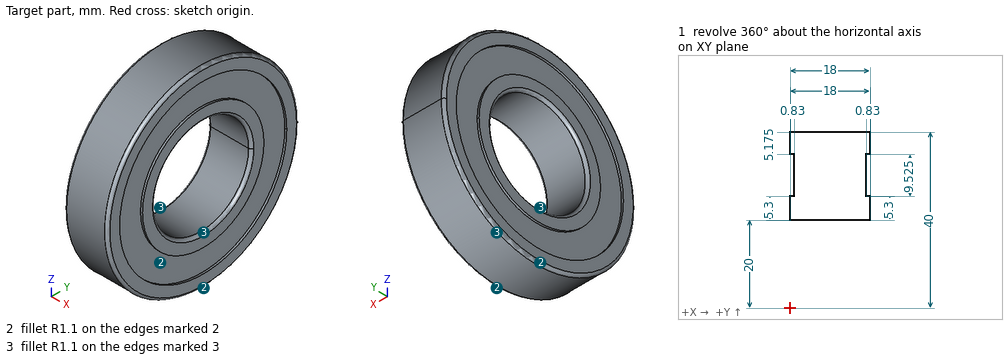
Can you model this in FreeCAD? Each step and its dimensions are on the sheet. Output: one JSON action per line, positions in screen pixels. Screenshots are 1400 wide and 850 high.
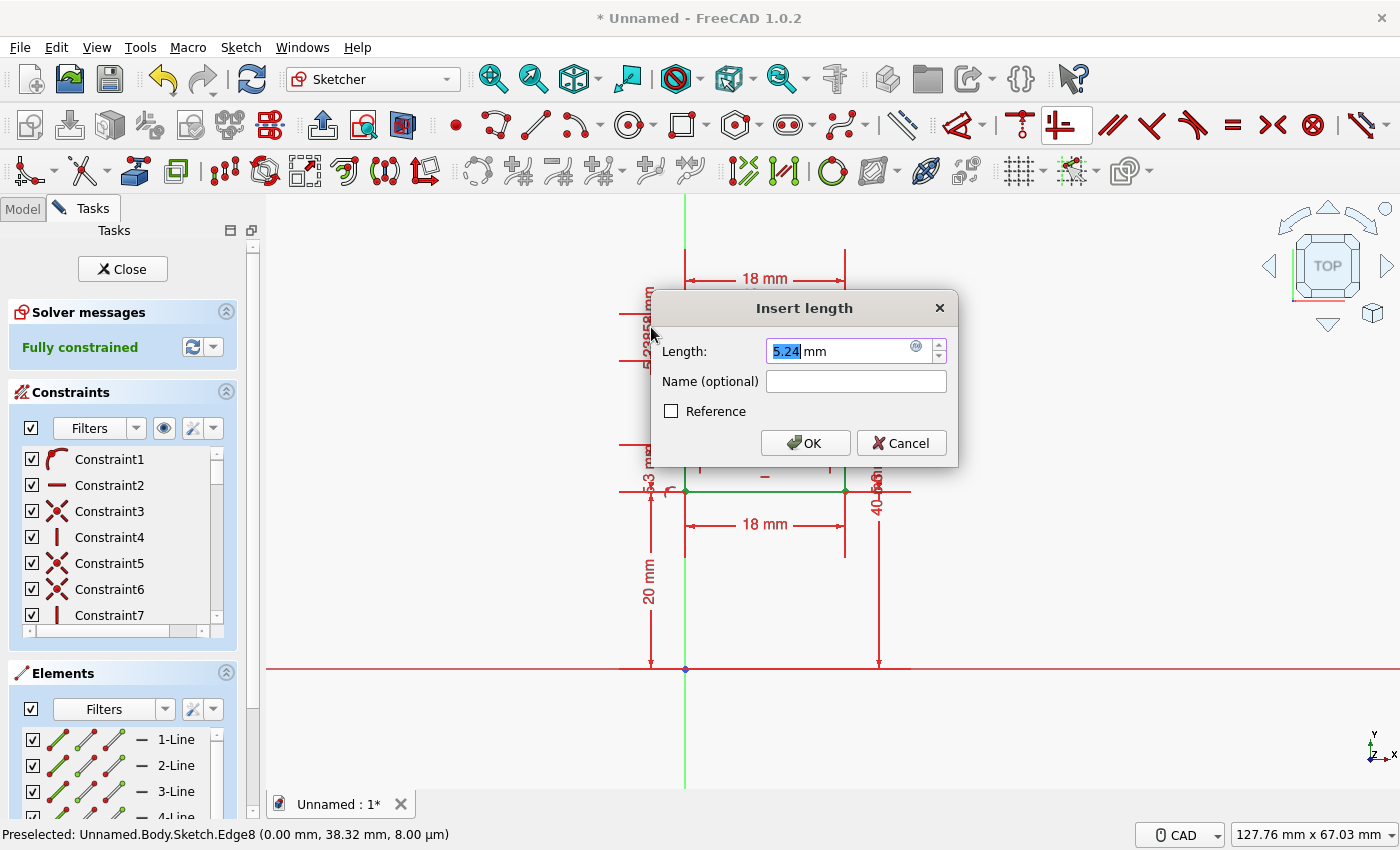
{"action": "type", "text": "5.175"}
{"action": "key", "text": "Return"}
{"action": "key", "text": "Escape"}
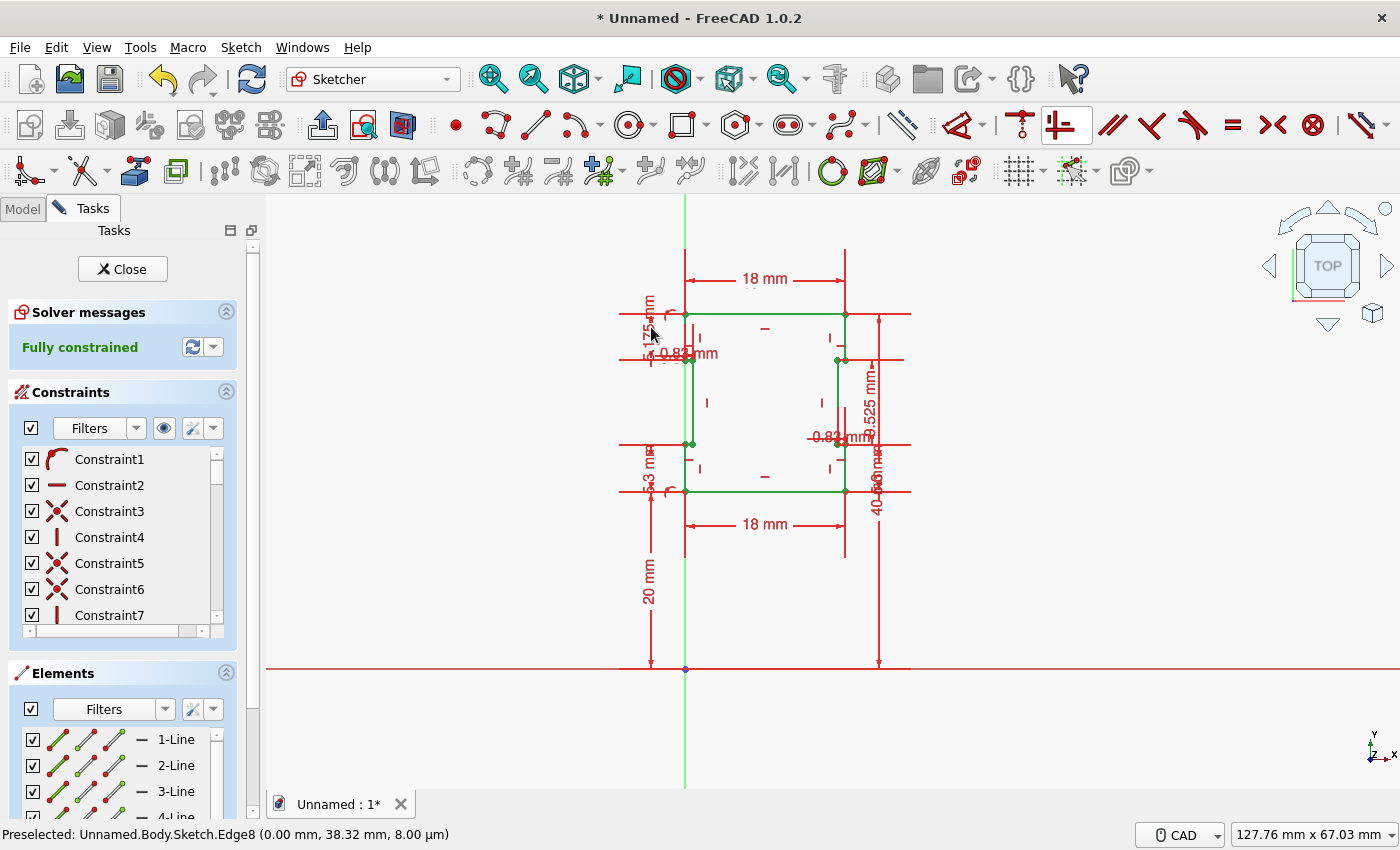
{"action": "left_click", "coordinate": [123, 269]}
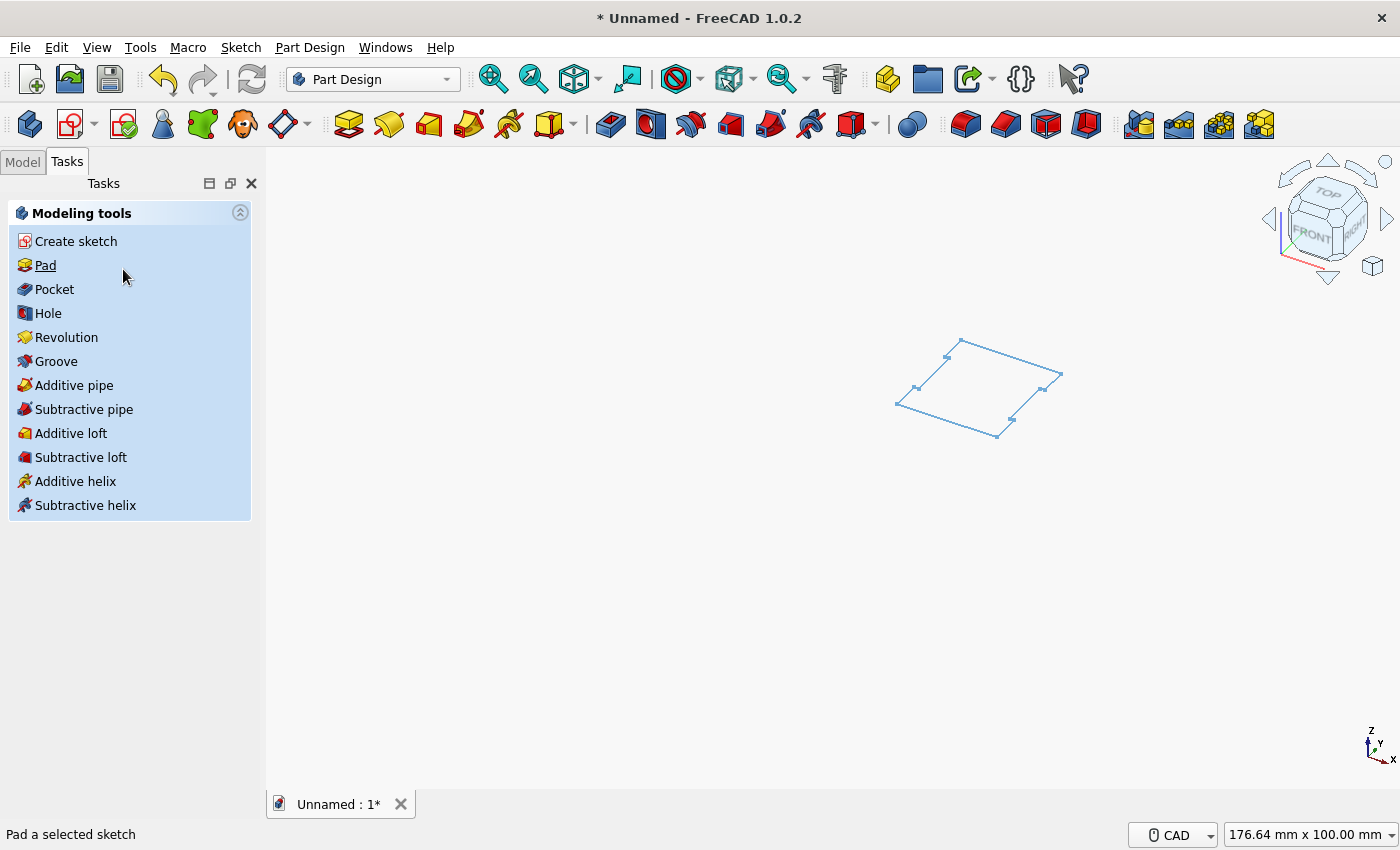
{"action": "left_click", "coordinate": [390, 124]}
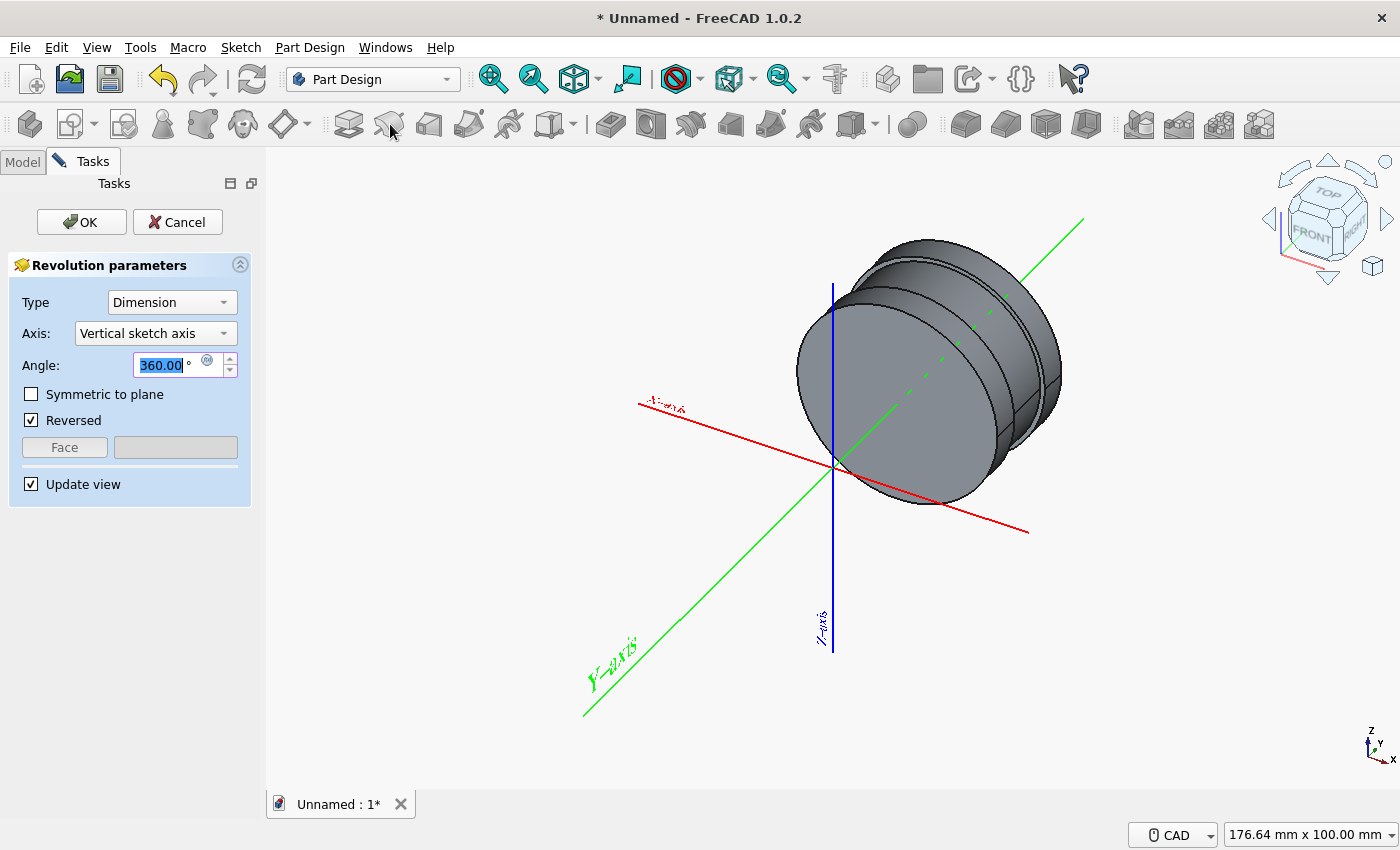
{"action": "left_click", "coordinate": [156, 334]}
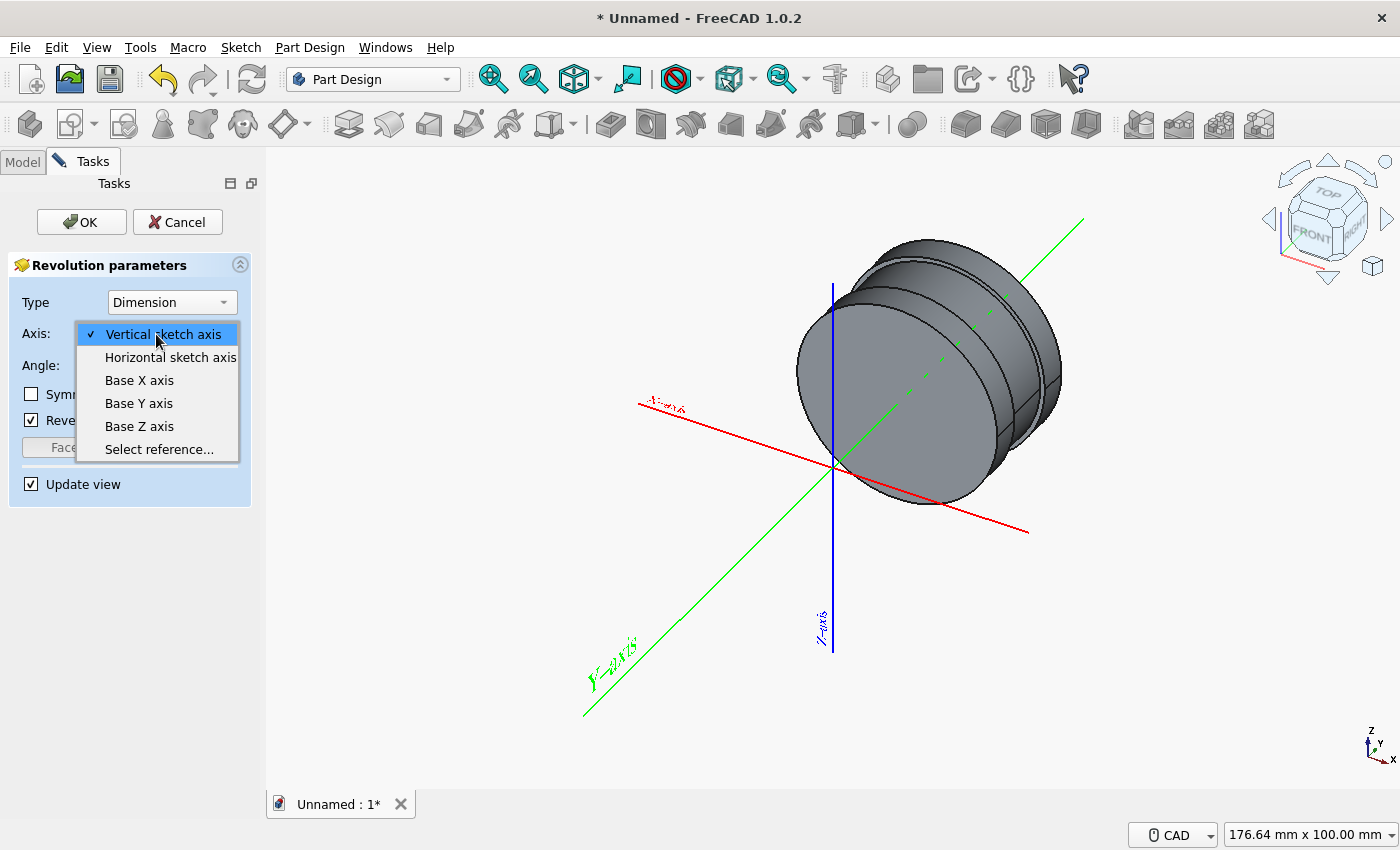
{"action": "left_click", "coordinate": [156, 358]}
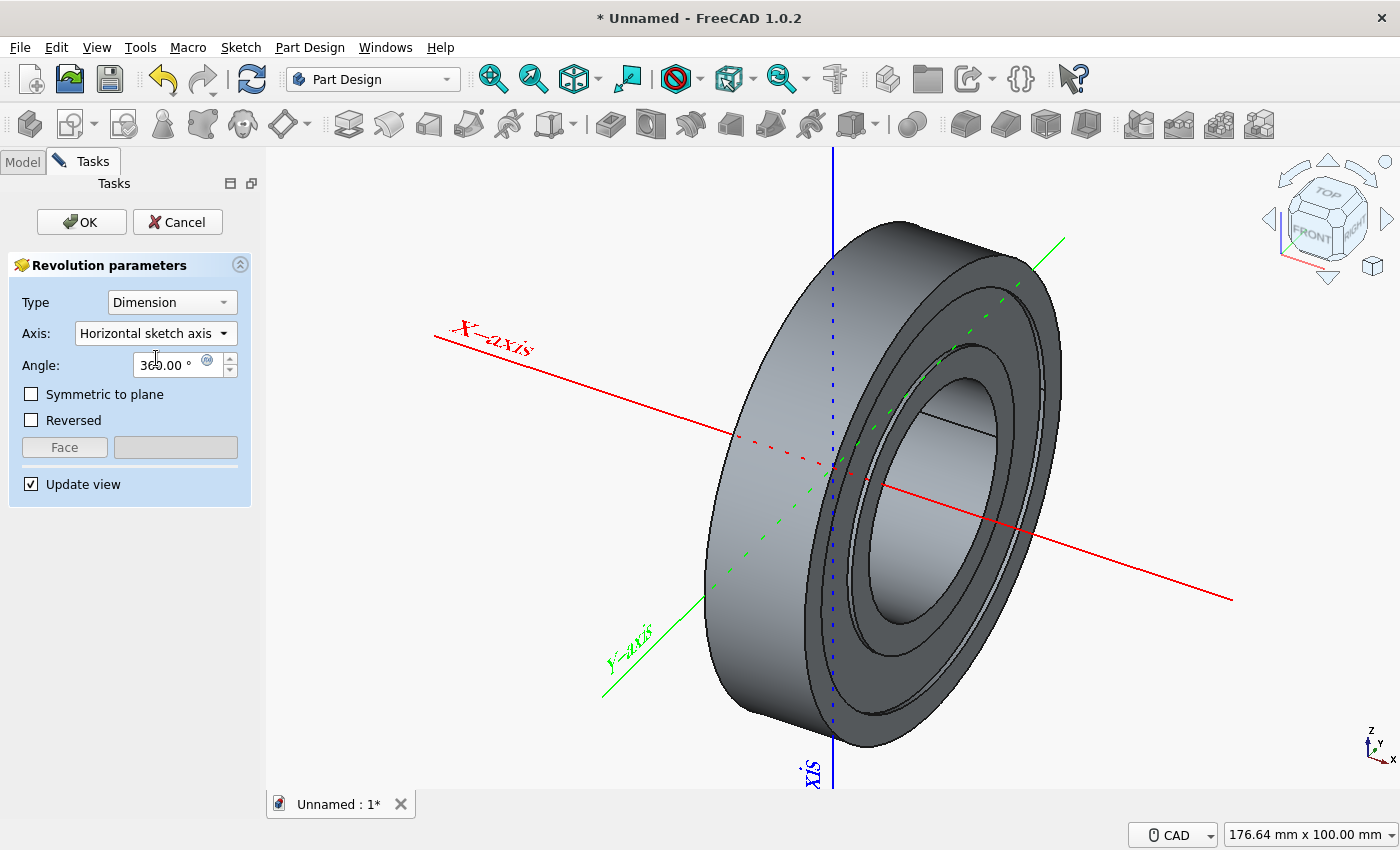
{"action": "left_click", "coordinate": [82, 222]}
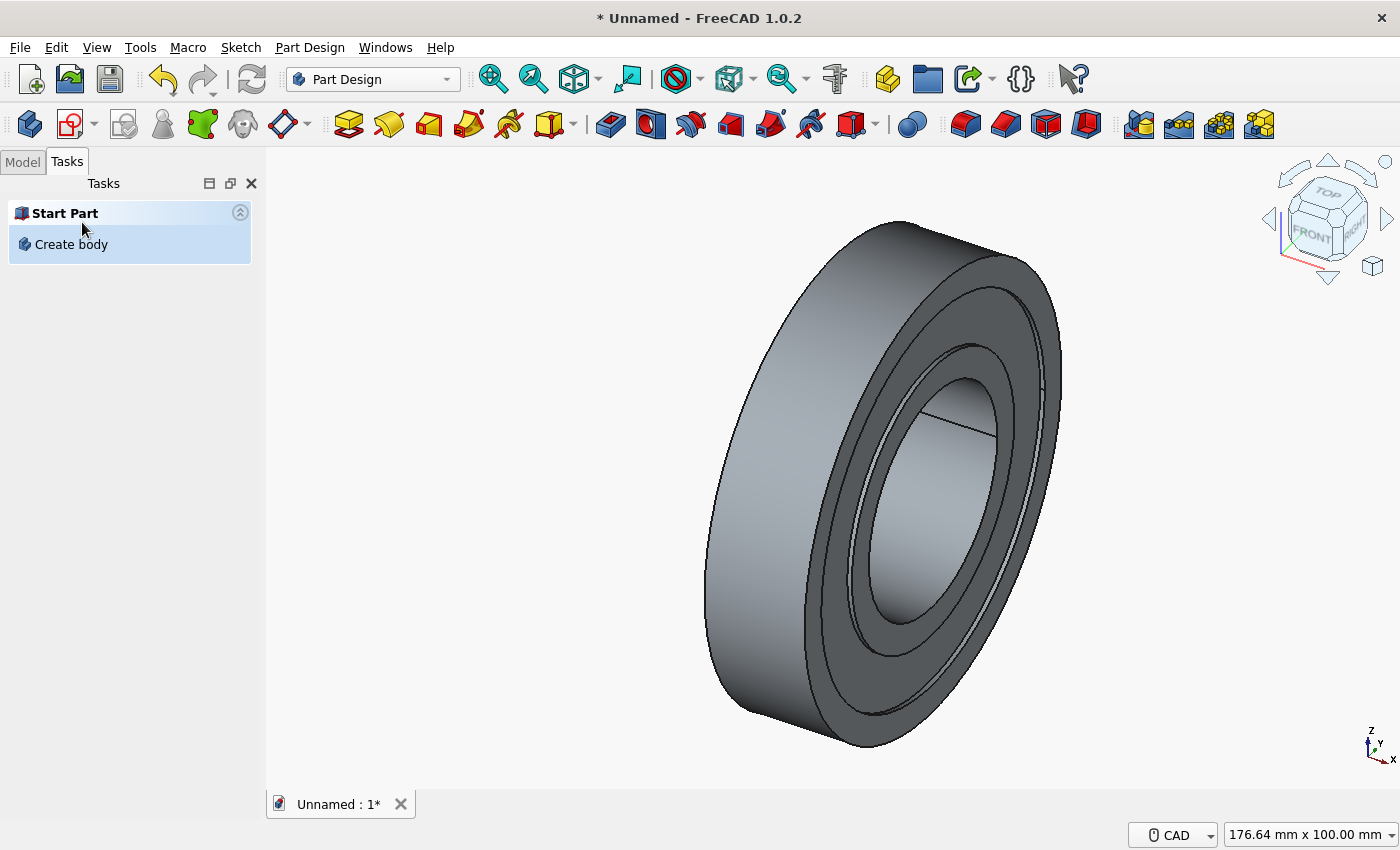
{"action": "left_click", "coordinate": [494, 80]}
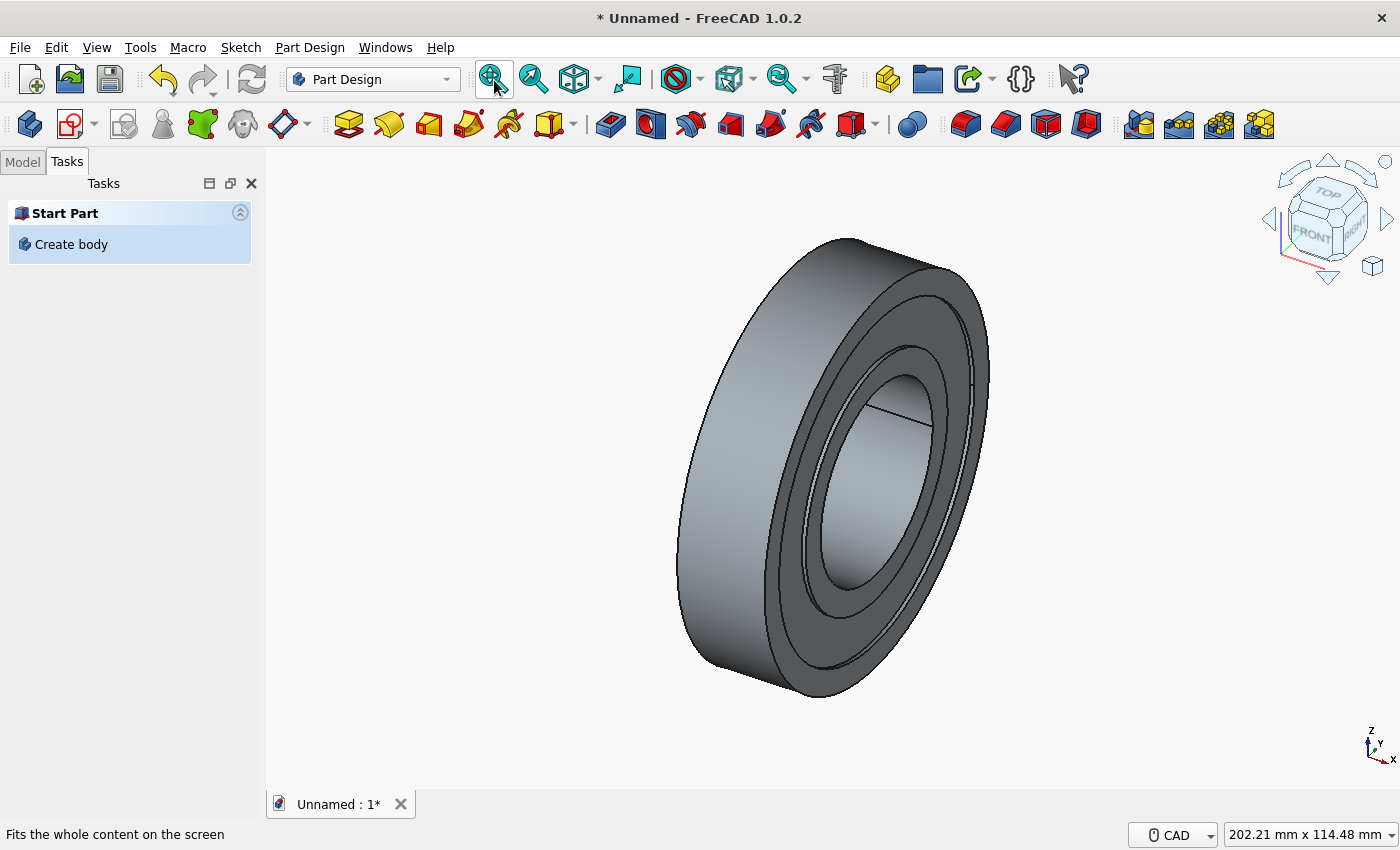
{"action": "left_click", "coordinate": [765, 593]}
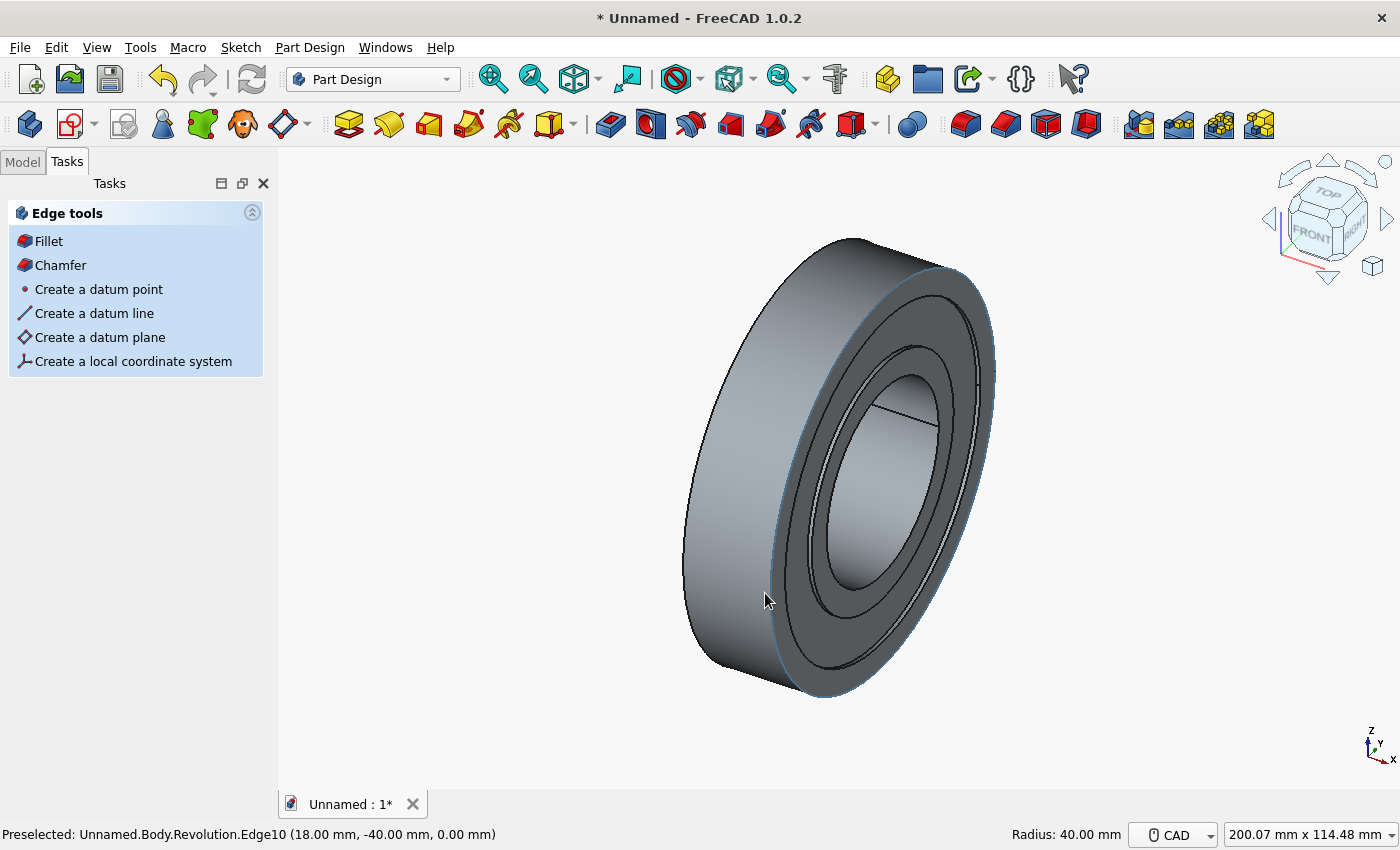
{"action": "key", "text": "0"}